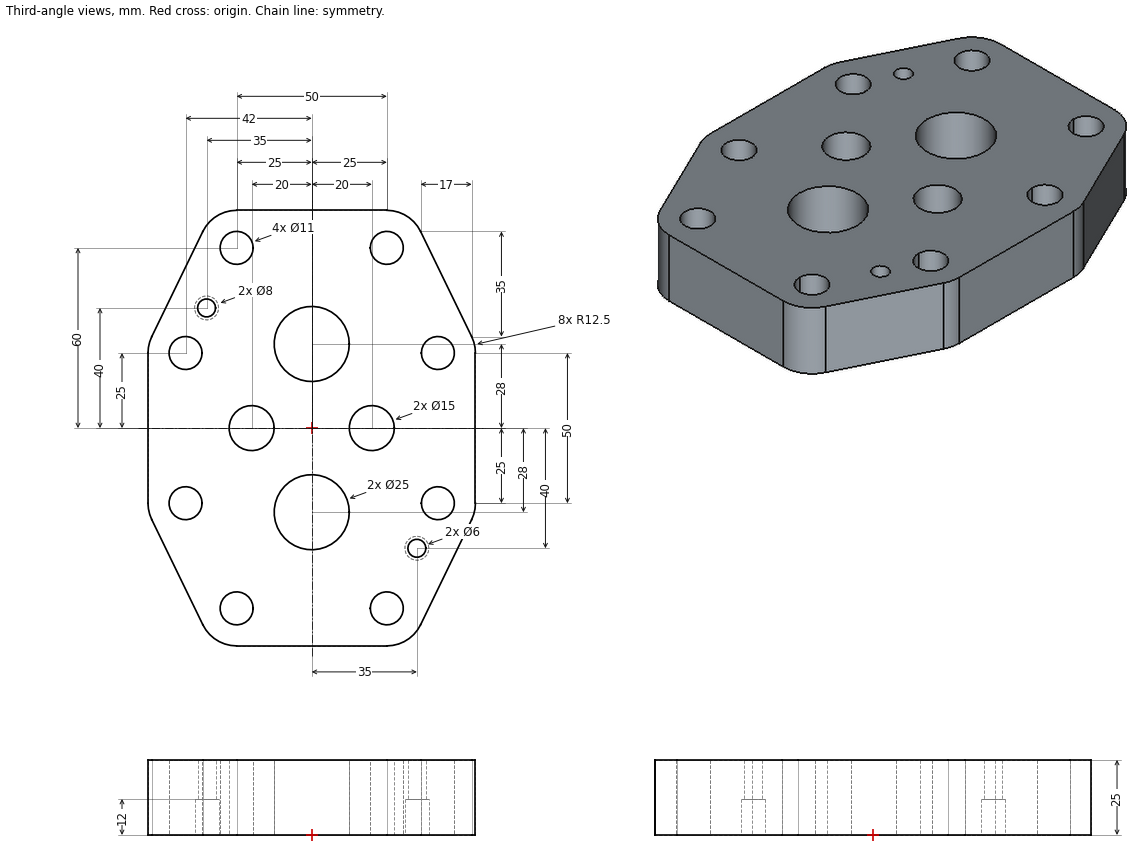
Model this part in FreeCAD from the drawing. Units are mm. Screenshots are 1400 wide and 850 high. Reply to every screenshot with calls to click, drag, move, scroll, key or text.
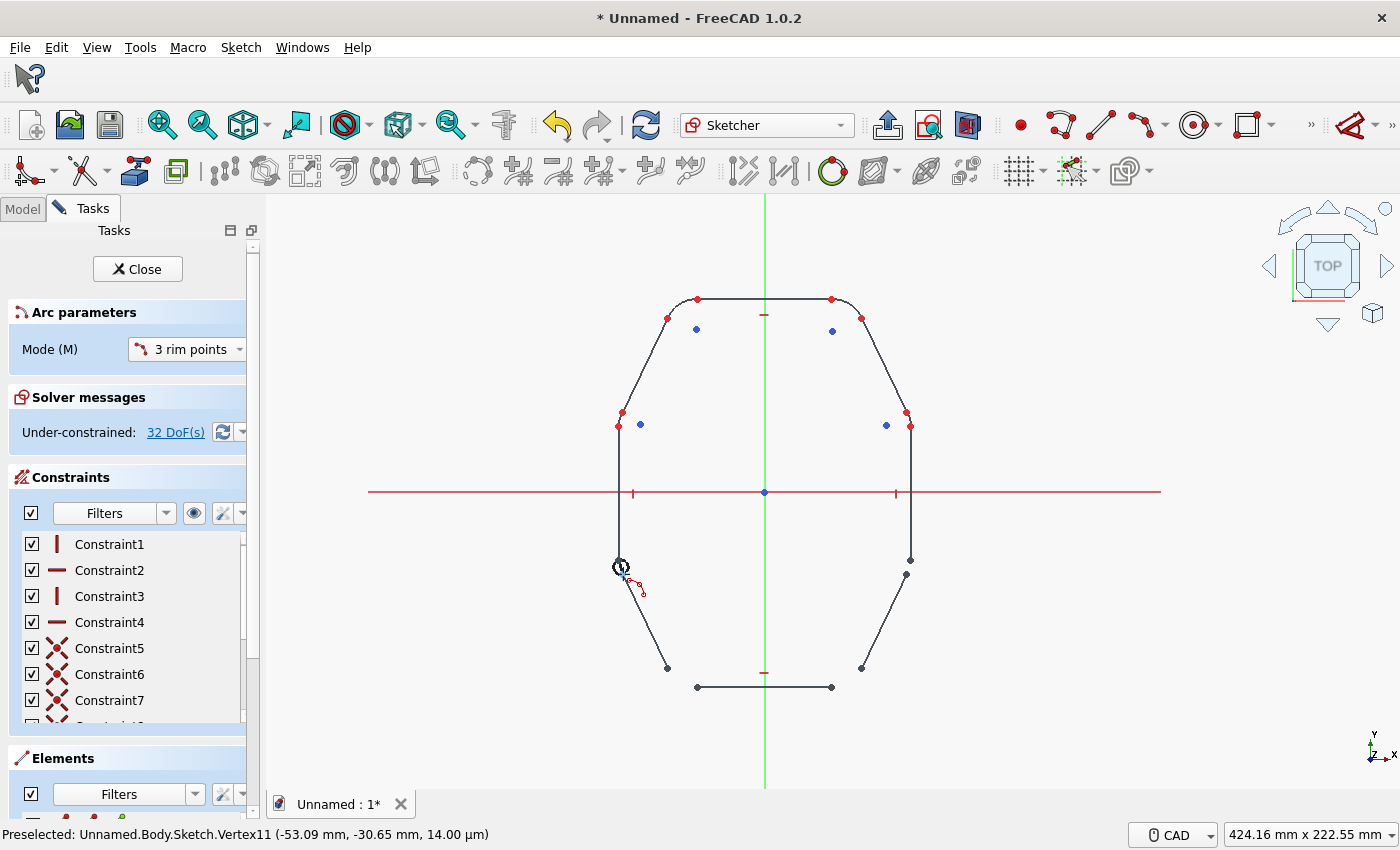
scroll(620, 567, up, 15)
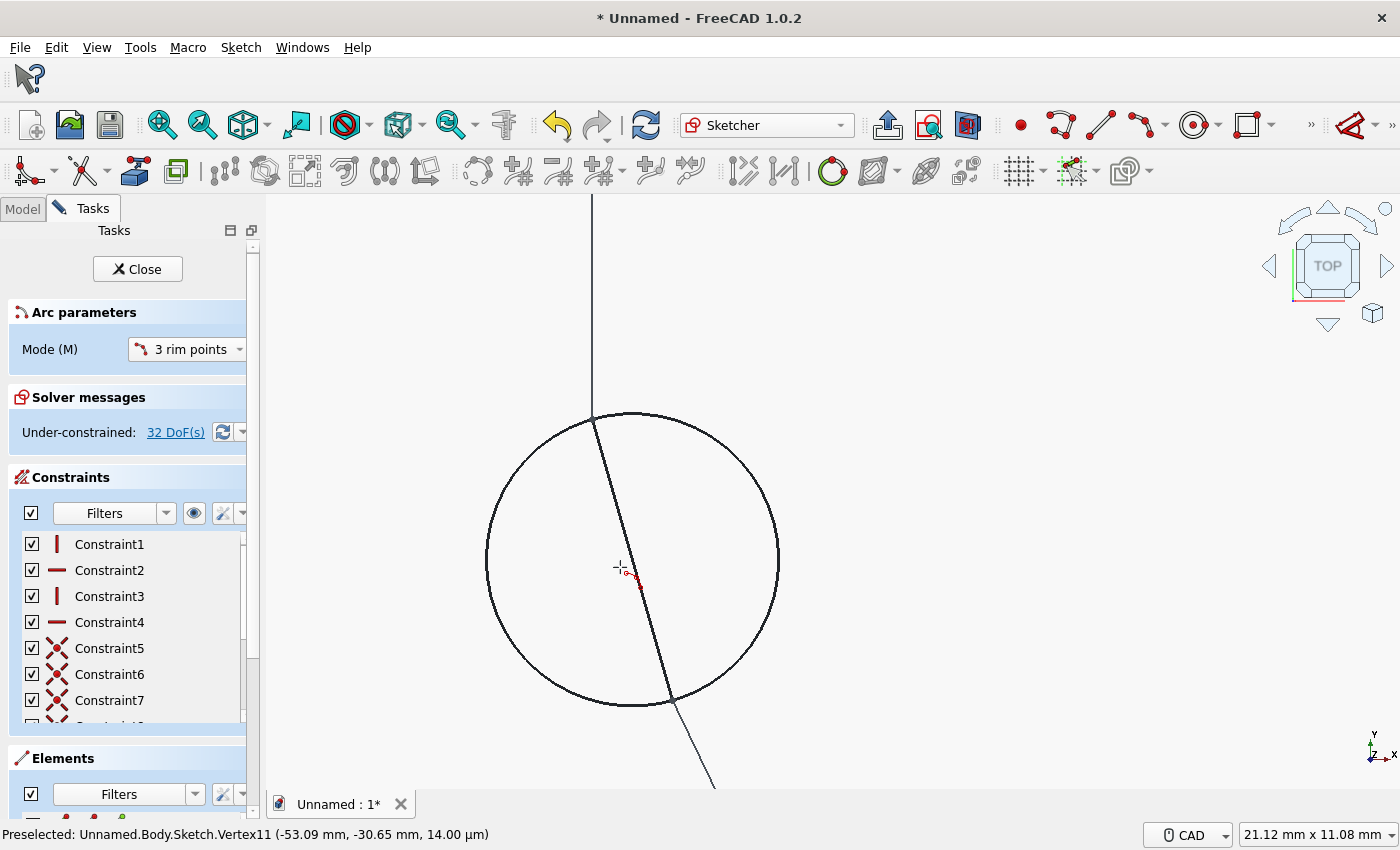
click(614, 547)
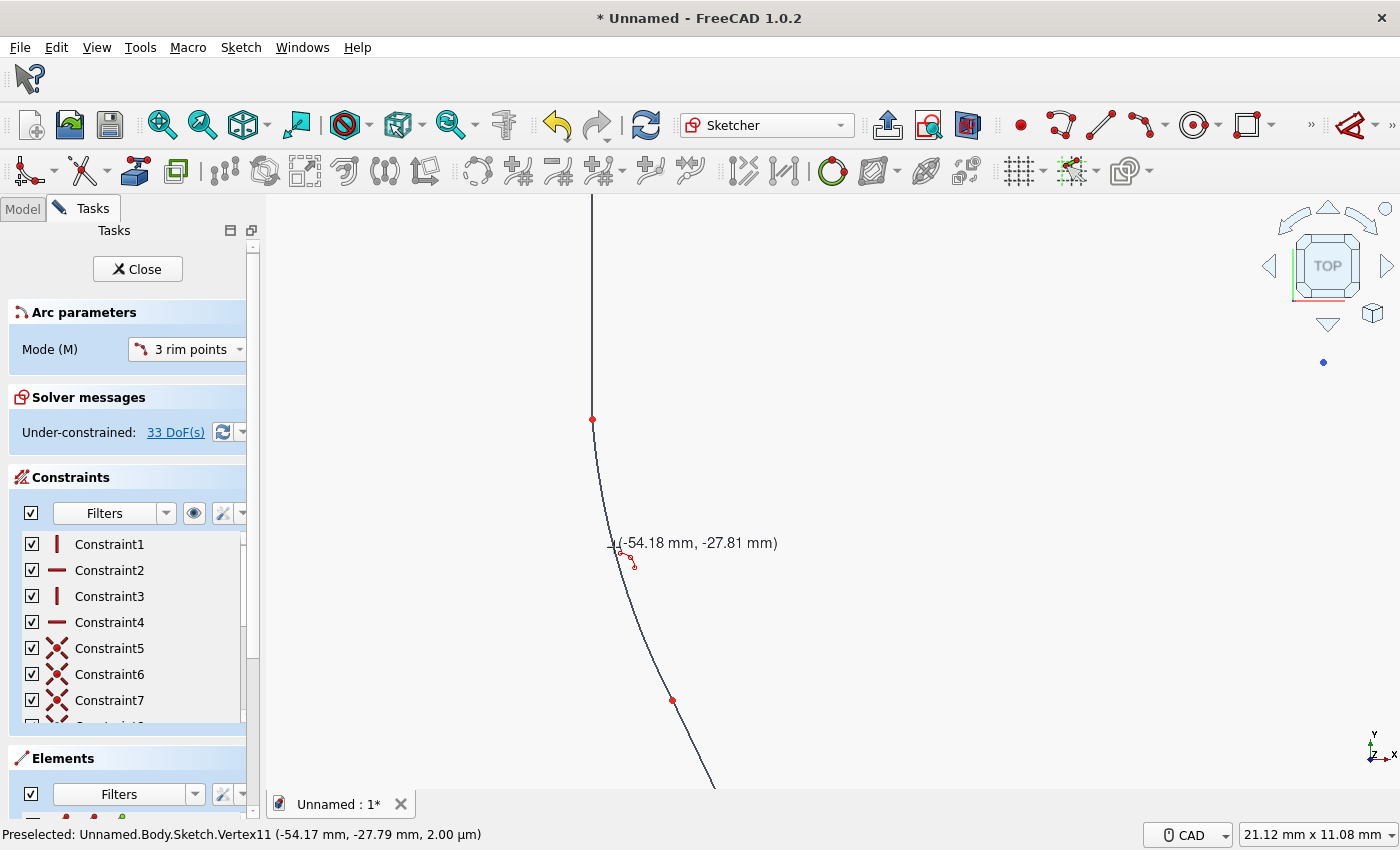
scroll(620, 567, down, 15)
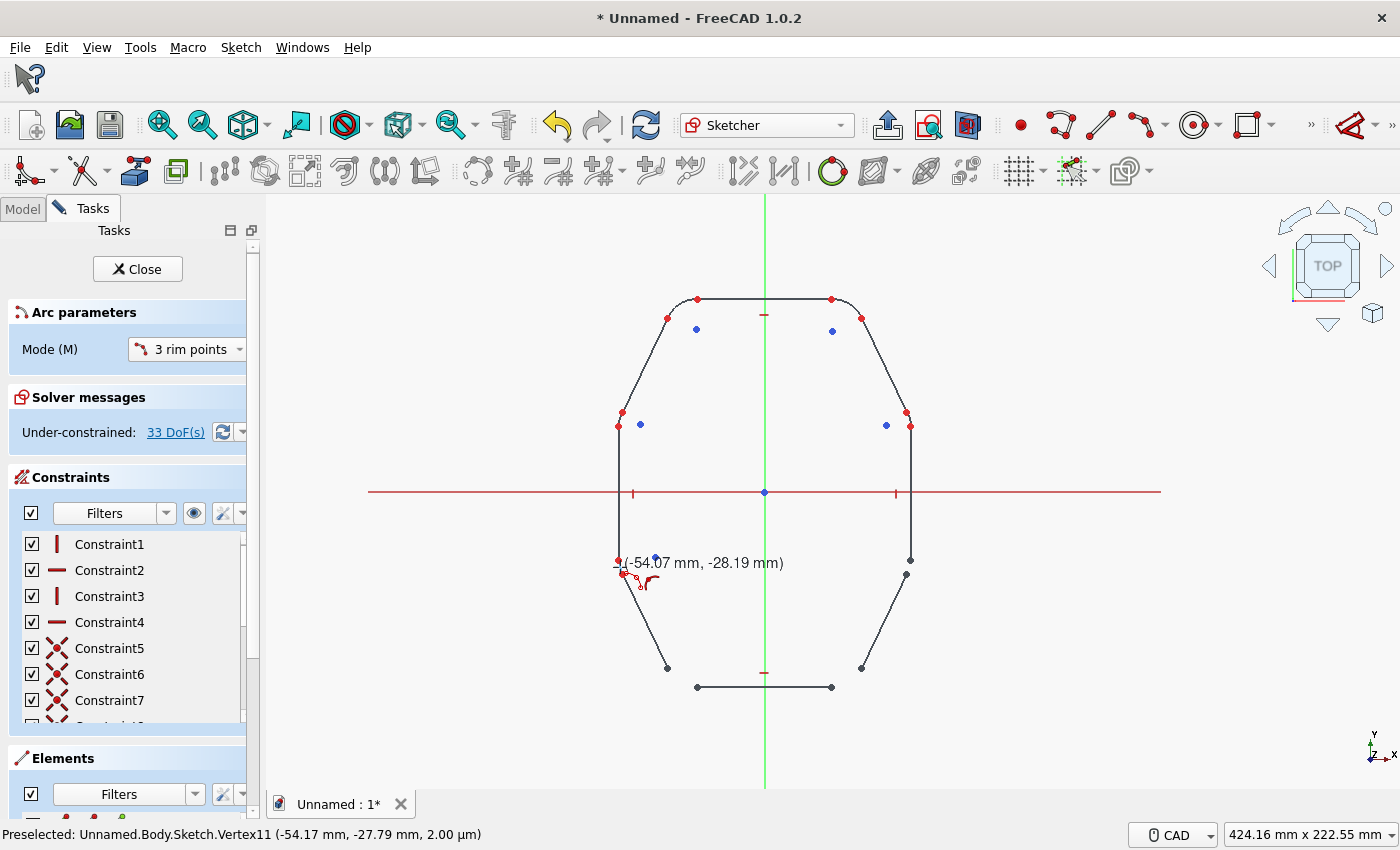
click(668, 668)
click(698, 687)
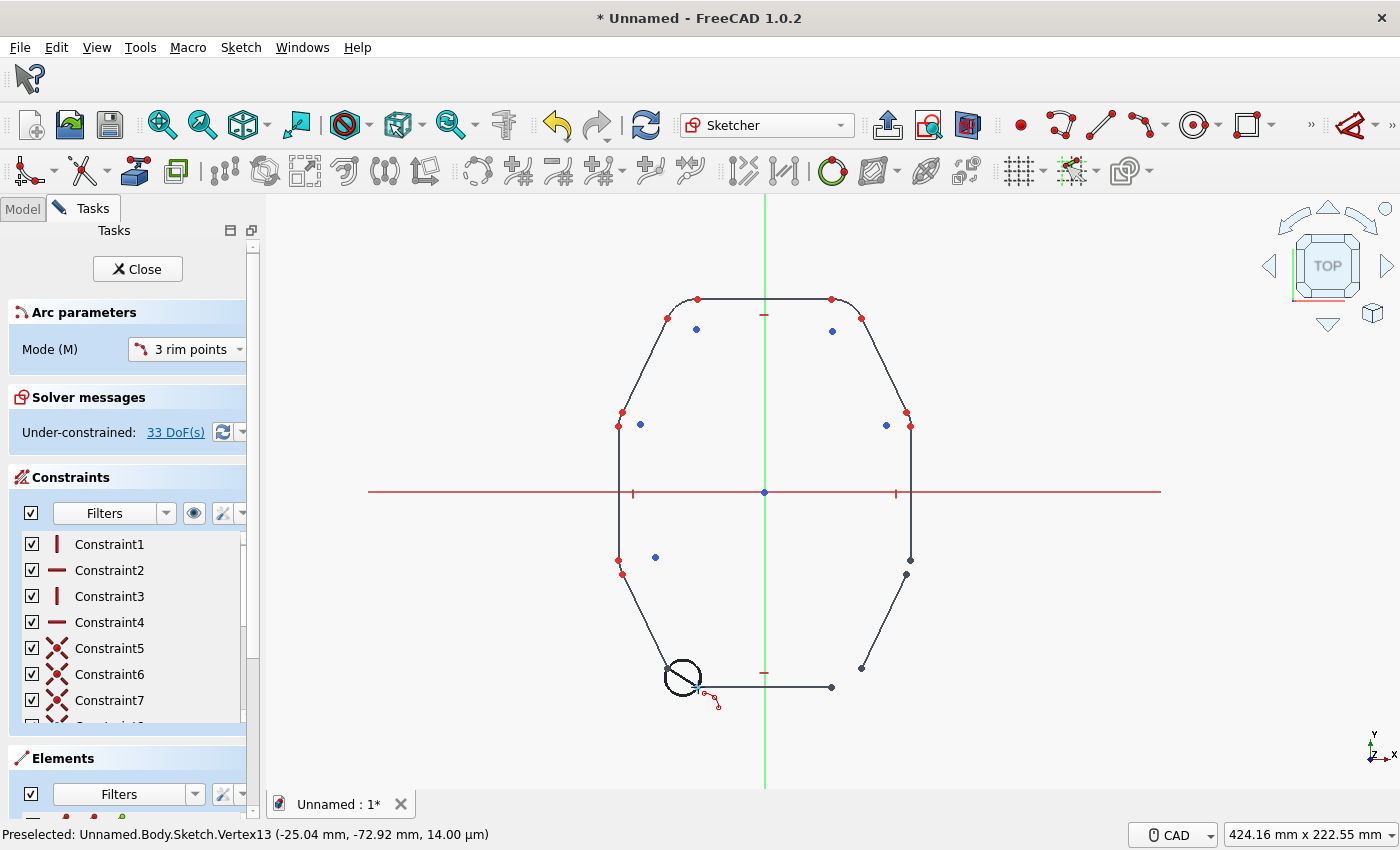
scroll(680, 681, up, 6)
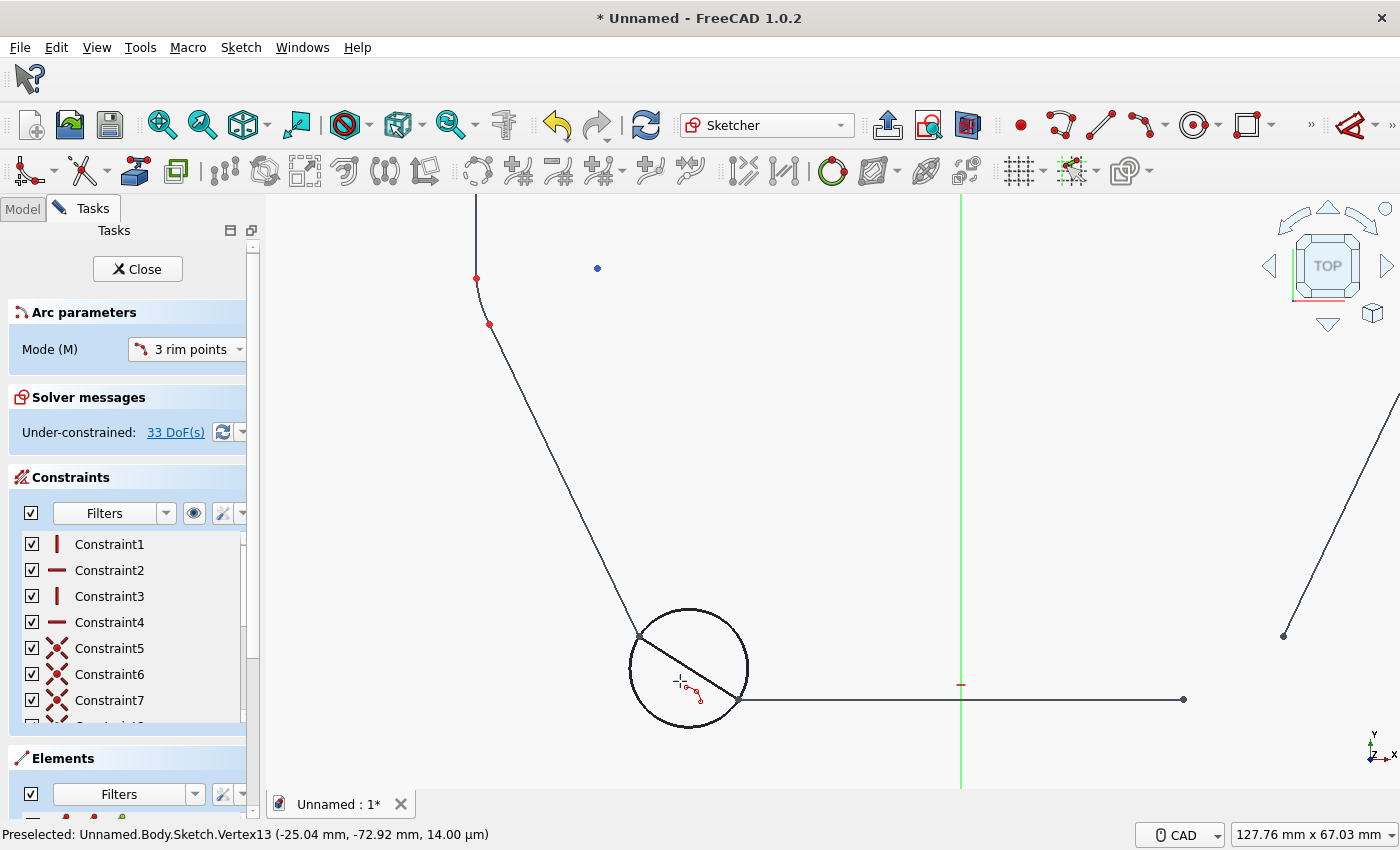
click(680, 679)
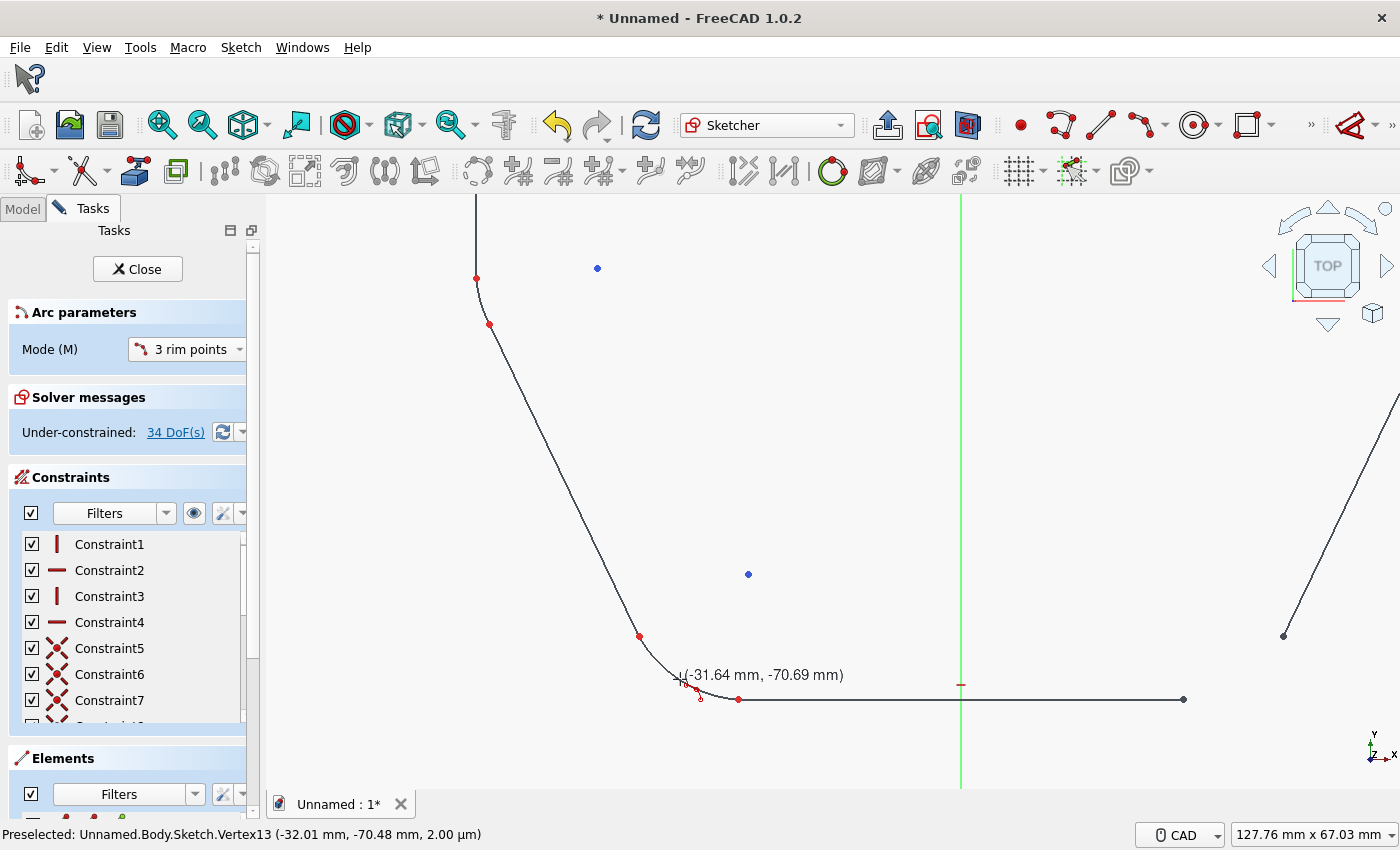
click(1184, 700)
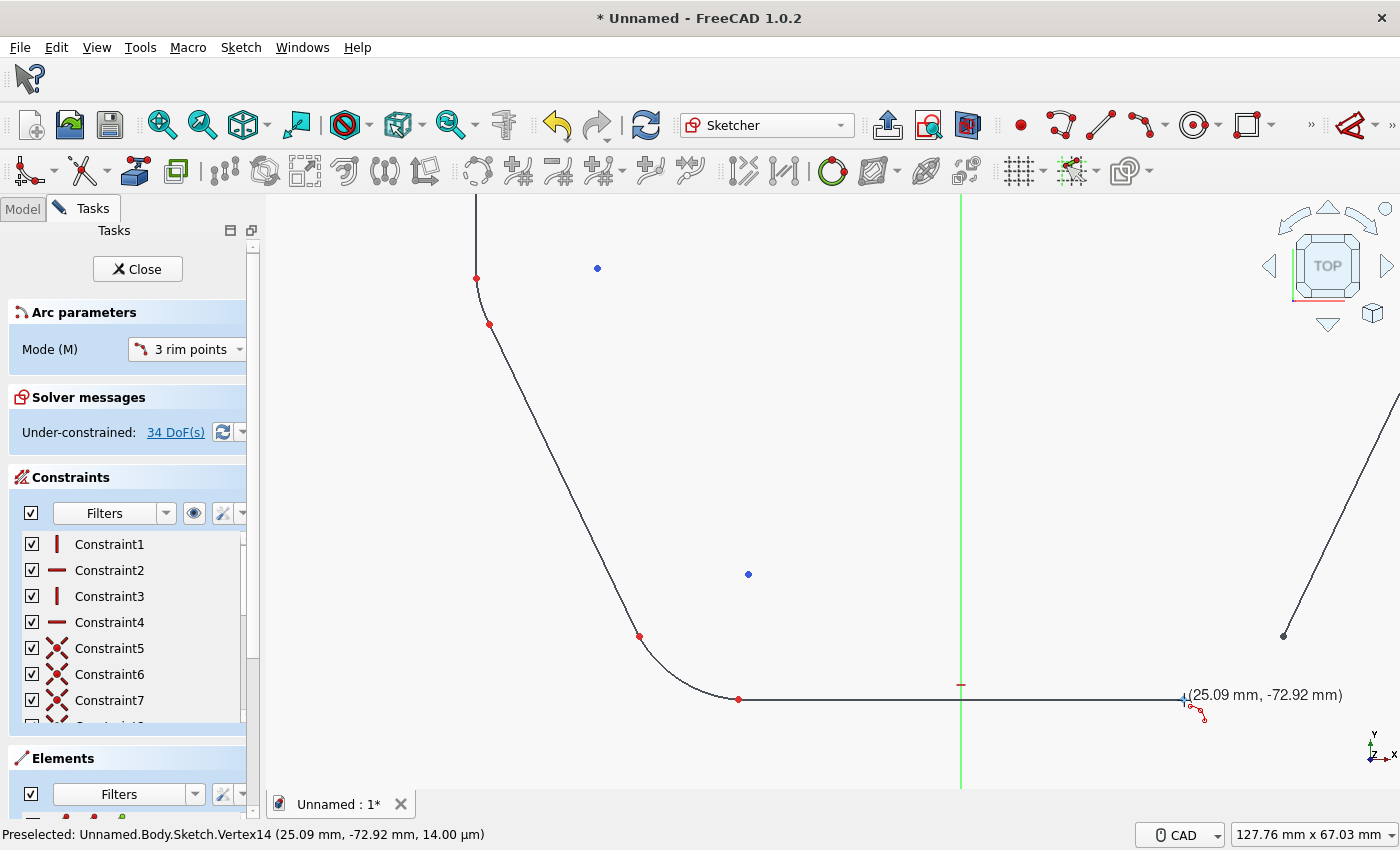
scroll(680, 681, down, 6)